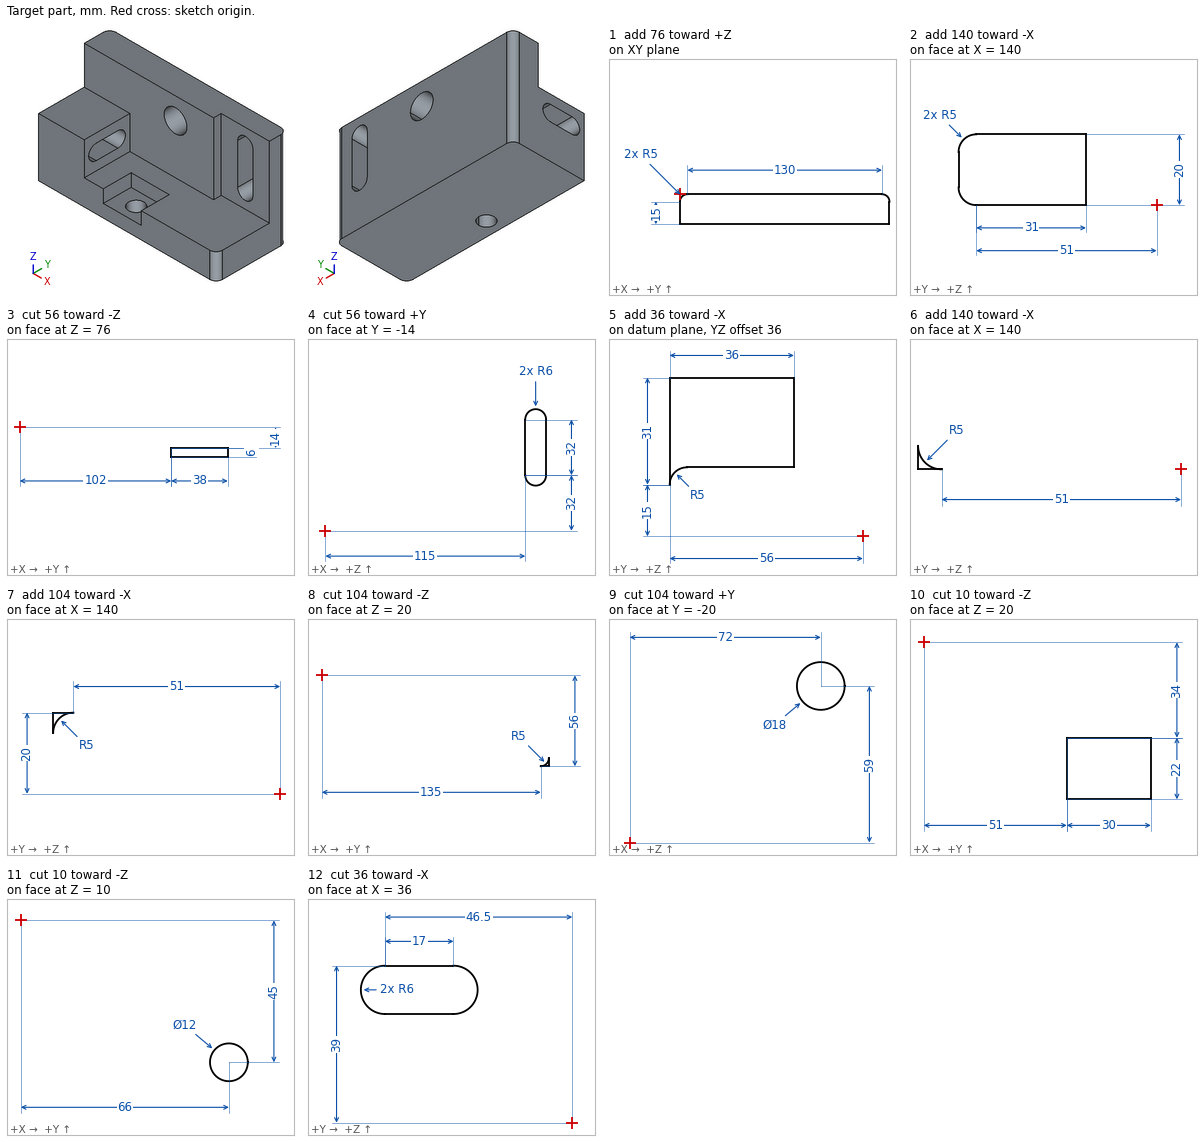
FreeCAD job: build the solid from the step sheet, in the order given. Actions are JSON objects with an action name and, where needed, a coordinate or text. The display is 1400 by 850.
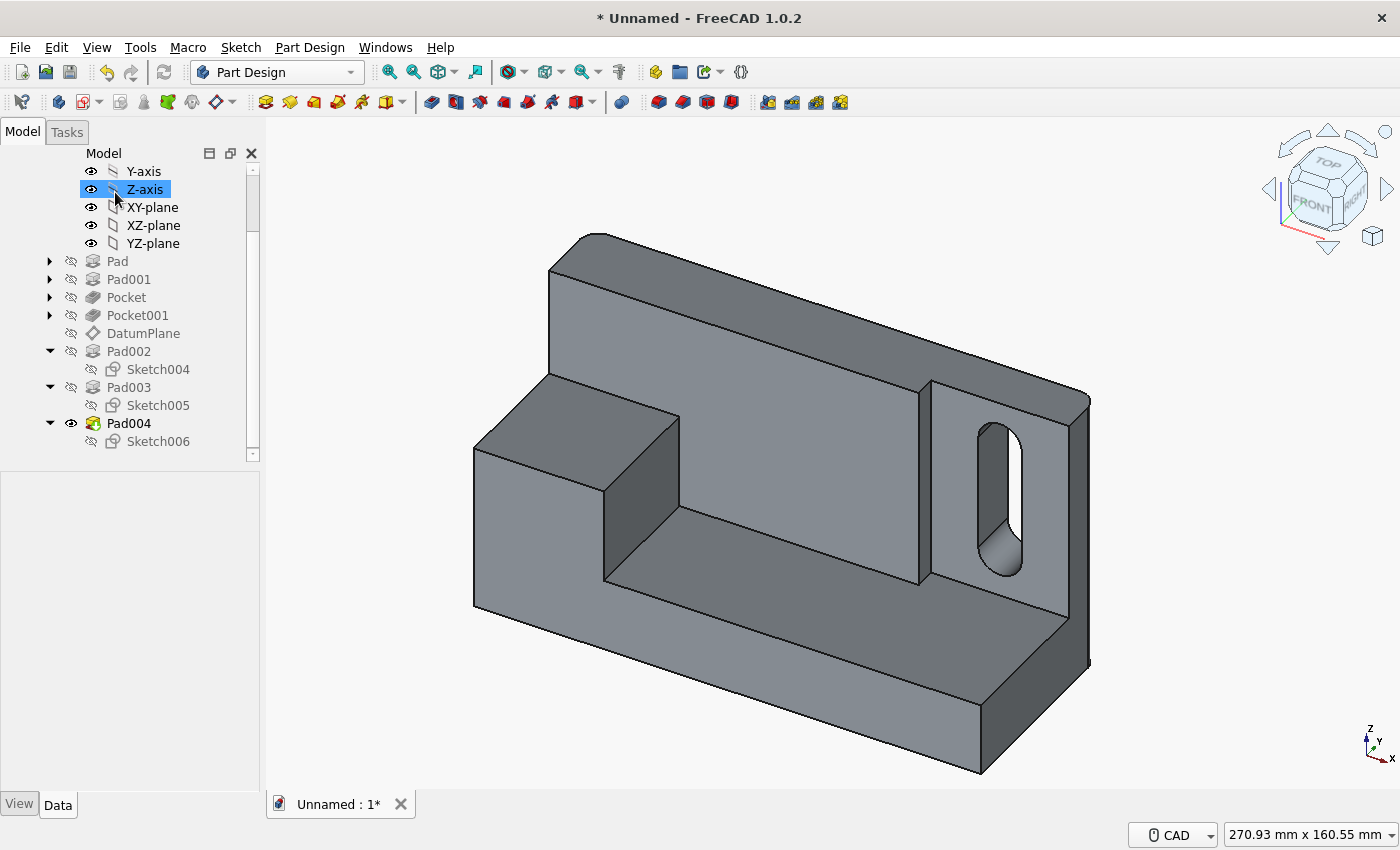
{"action": "left_click", "coordinate": [944, 634]}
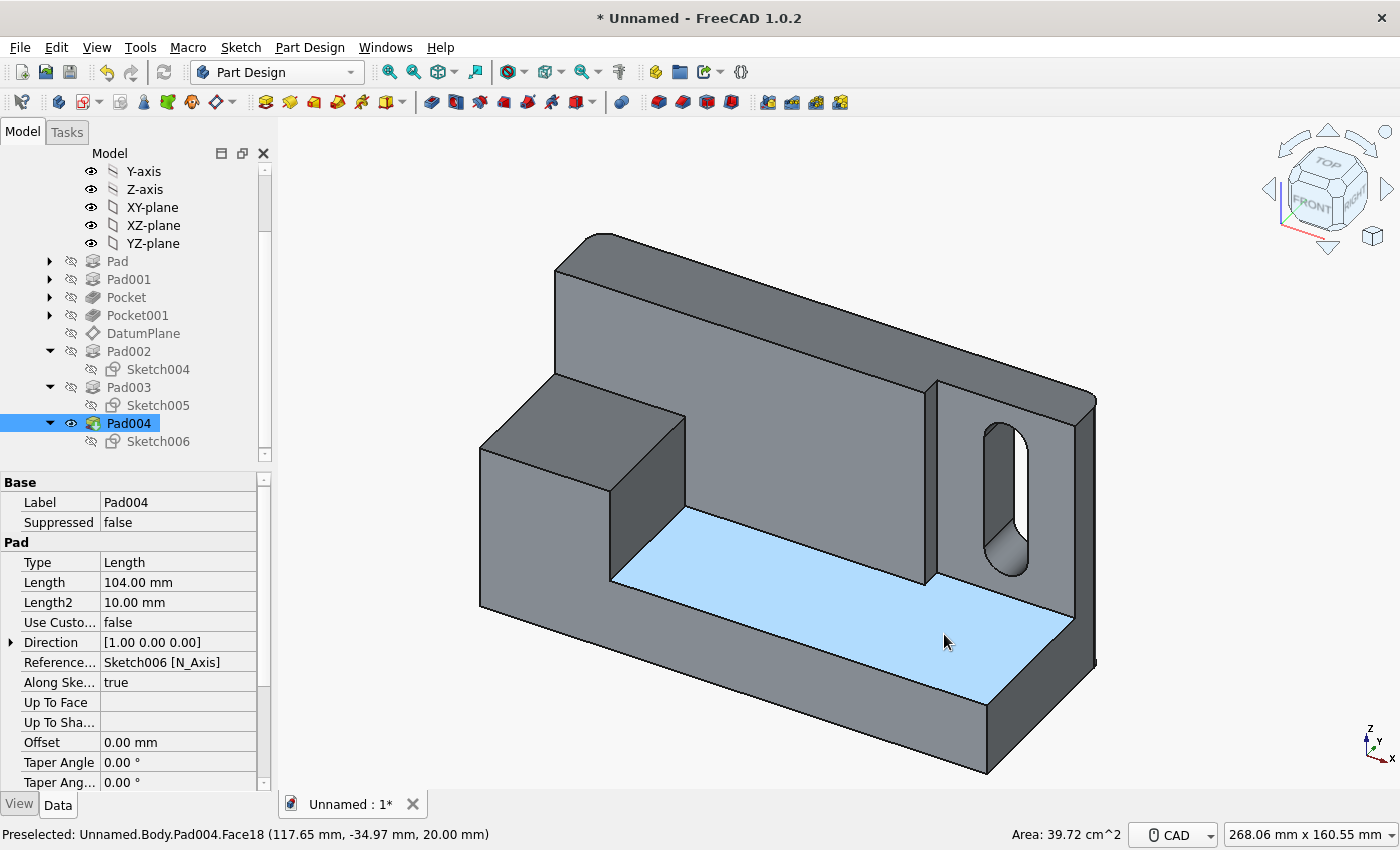
{"action": "left_click", "coordinate": [84, 102]}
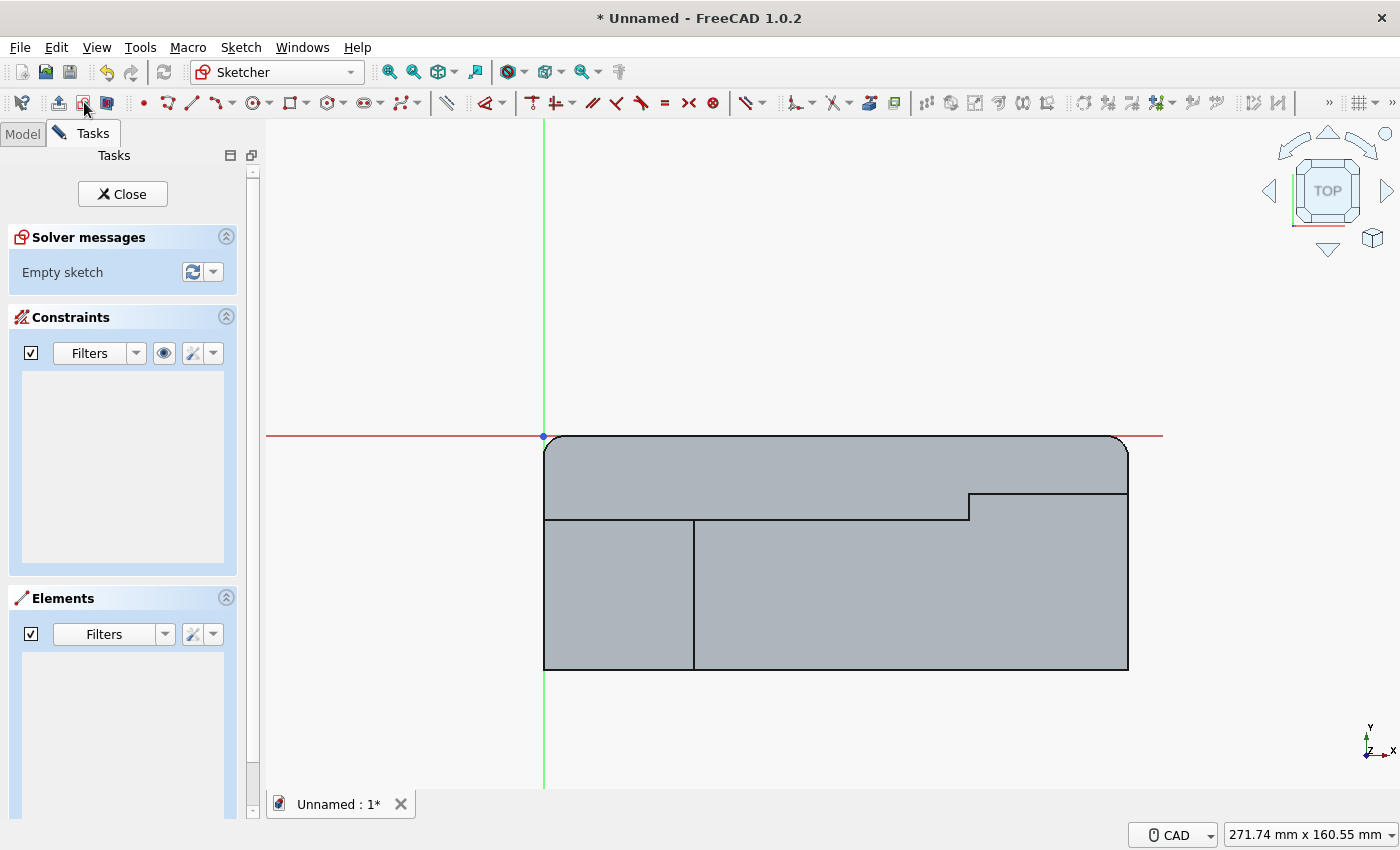
{"action": "scroll", "coordinate": [1136, 670], "scroll_direction": "up", "scroll_amount": 15}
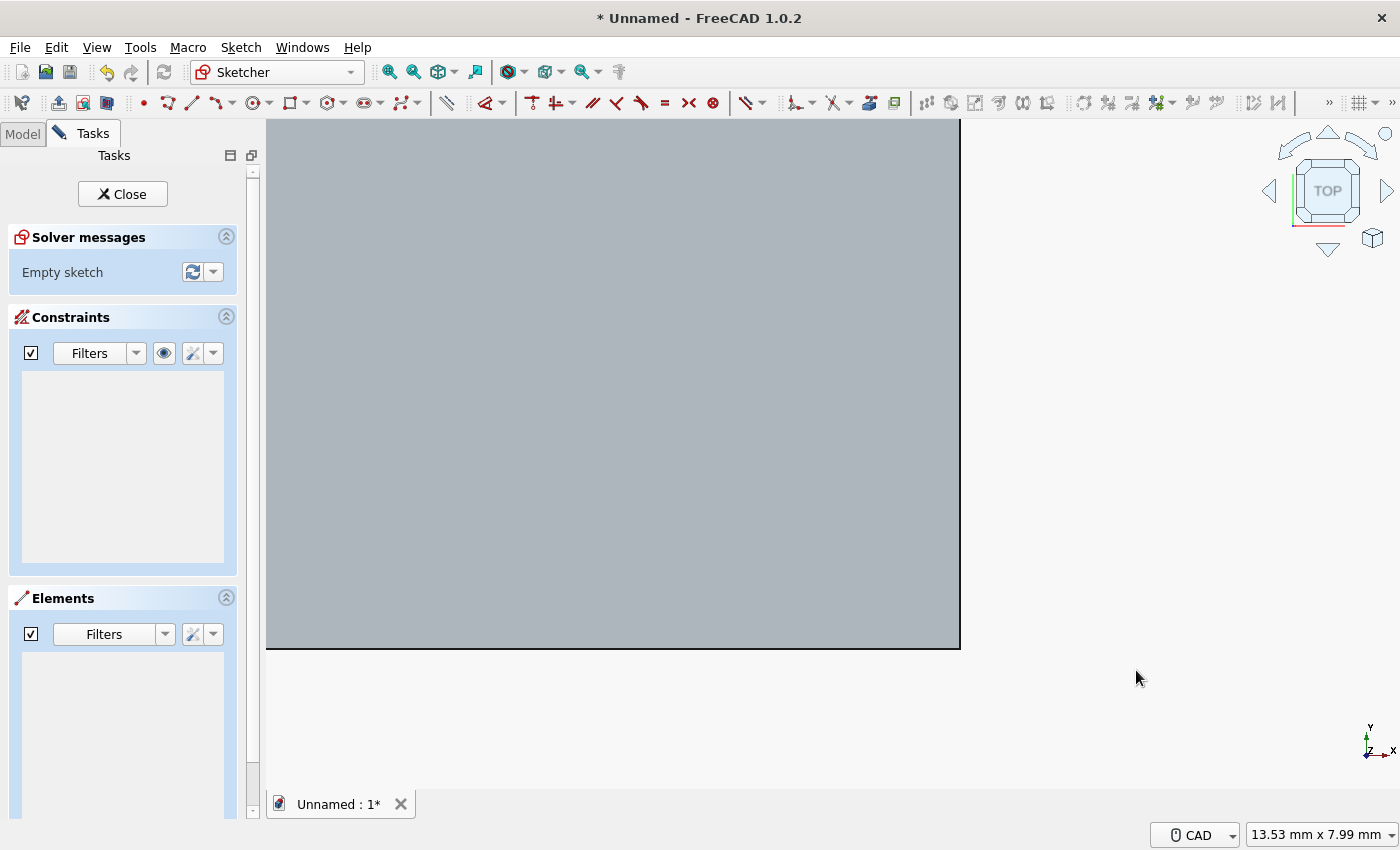
{"action": "left_click", "coordinate": [168, 104]}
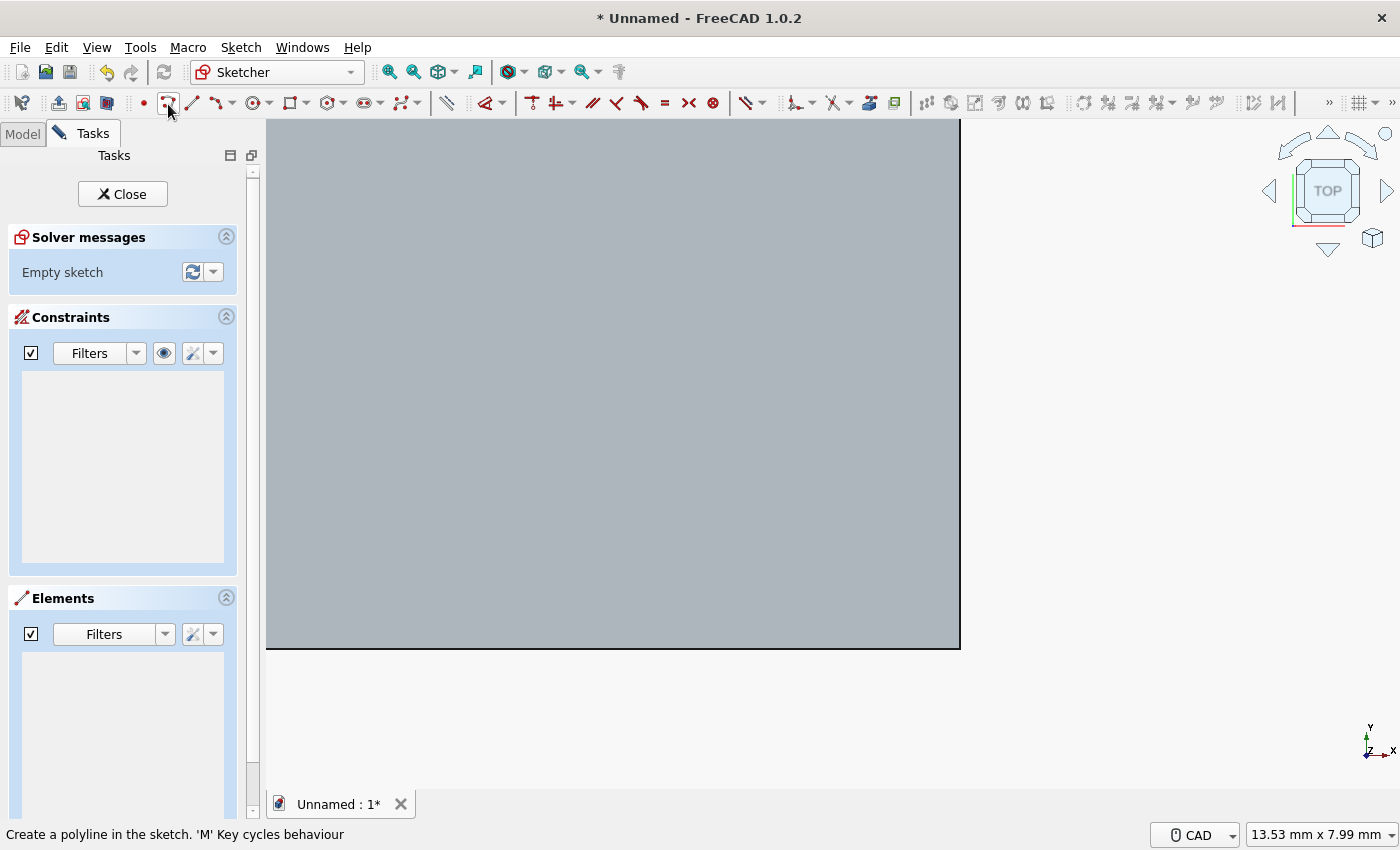
{"action": "left_click", "coordinate": [541, 649]}
{"action": "left_click", "coordinate": [960, 649]}
{"action": "left_click", "coordinate": [960, 230]}
{"action": "right_click", "coordinate": [960, 230]}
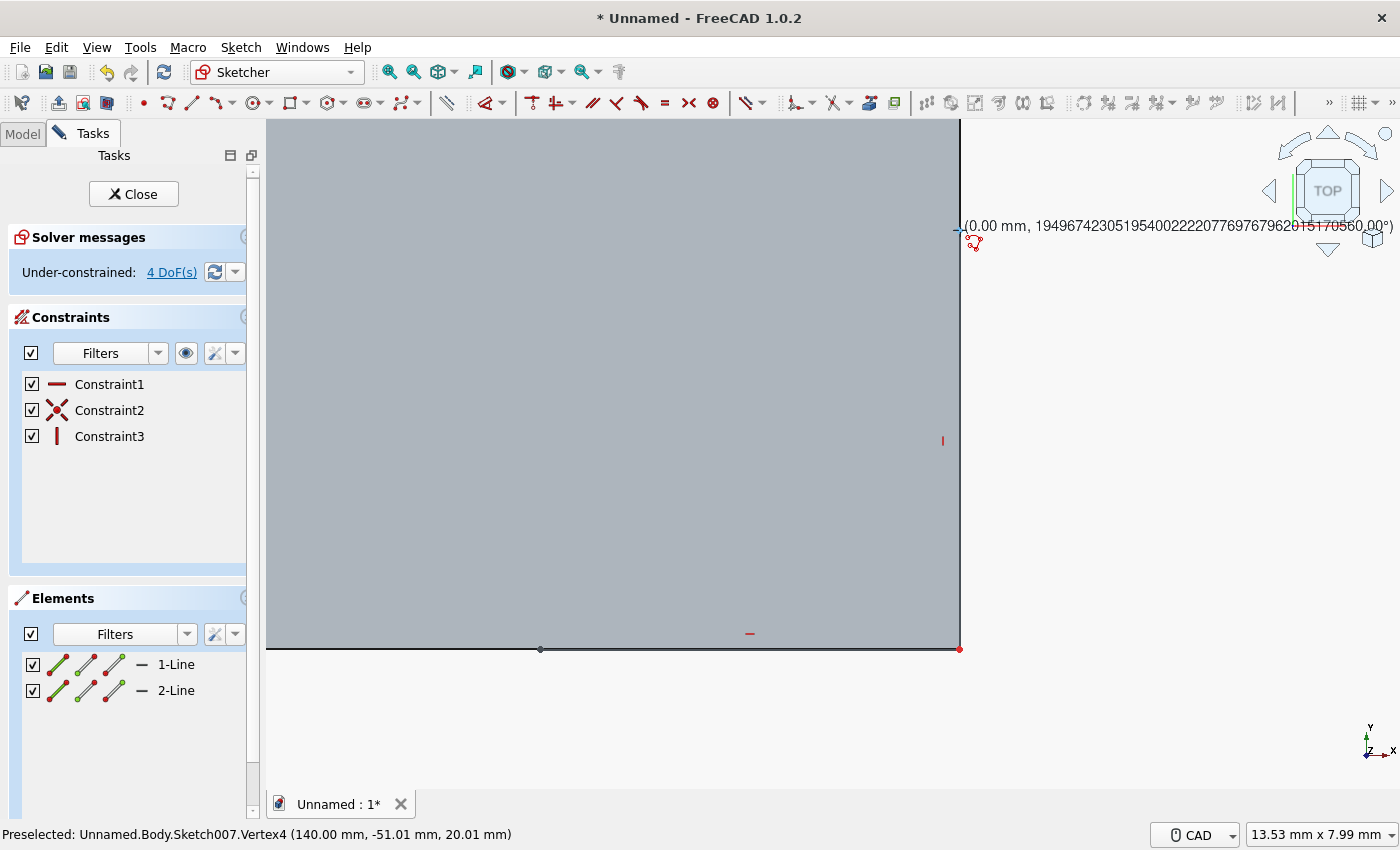
{"action": "left_click", "coordinate": [216, 104]}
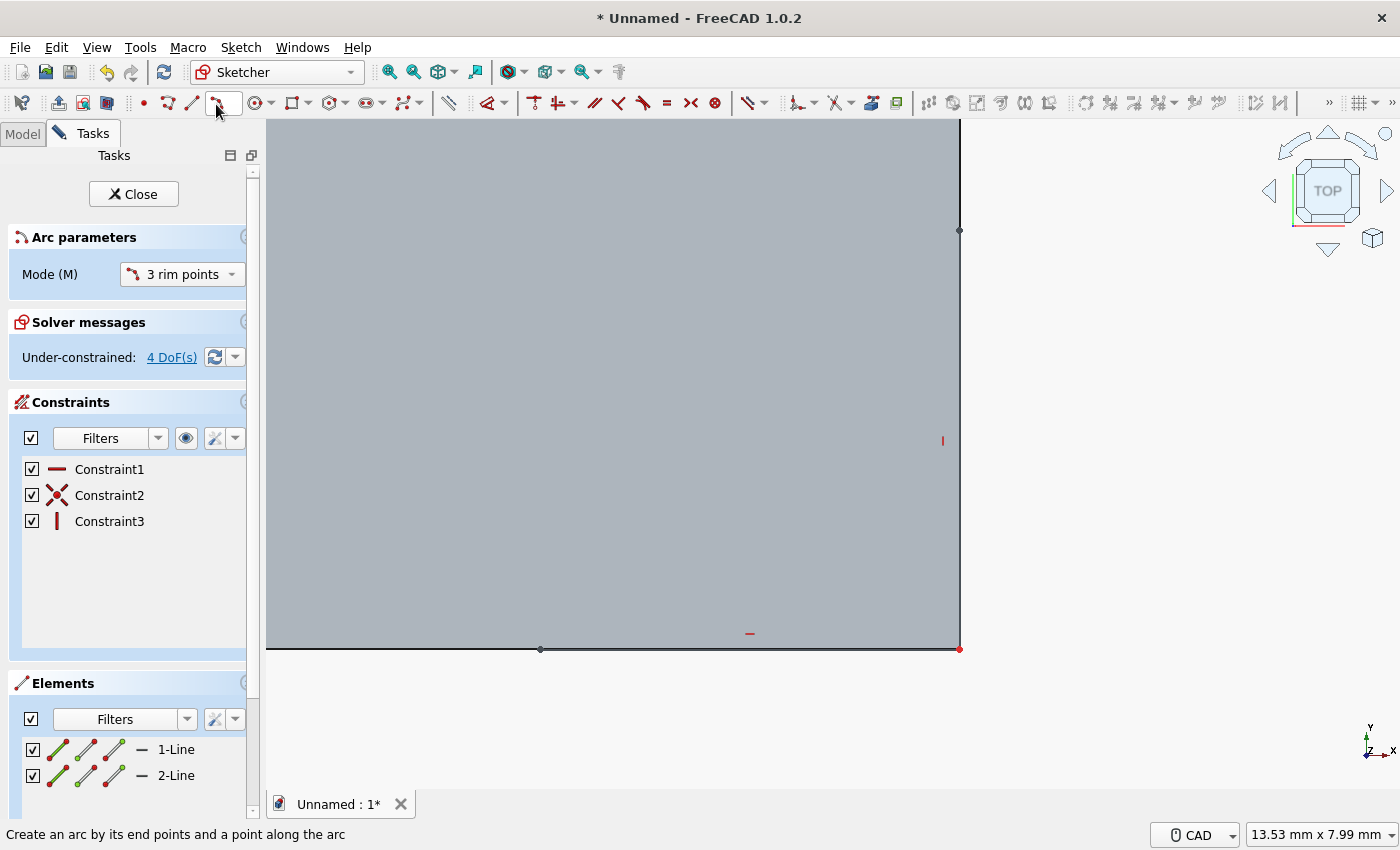
{"action": "left_click", "coordinate": [960, 231]}
{"action": "left_click", "coordinate": [541, 650]}
{"action": "left_click", "coordinate": [837, 526]}
{"action": "key", "text": "Escape"}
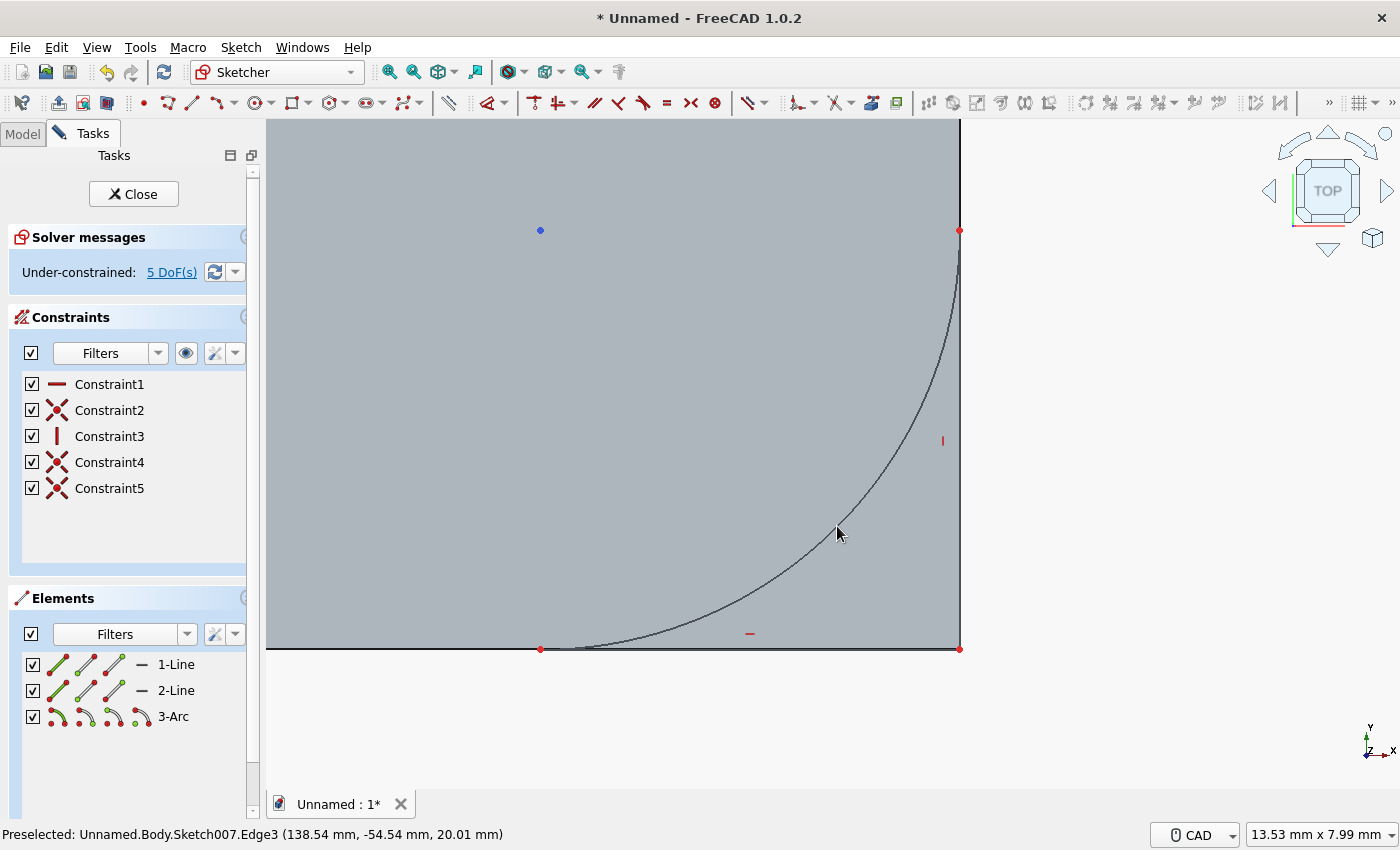
{"action": "left_click", "coordinate": [667, 650]}